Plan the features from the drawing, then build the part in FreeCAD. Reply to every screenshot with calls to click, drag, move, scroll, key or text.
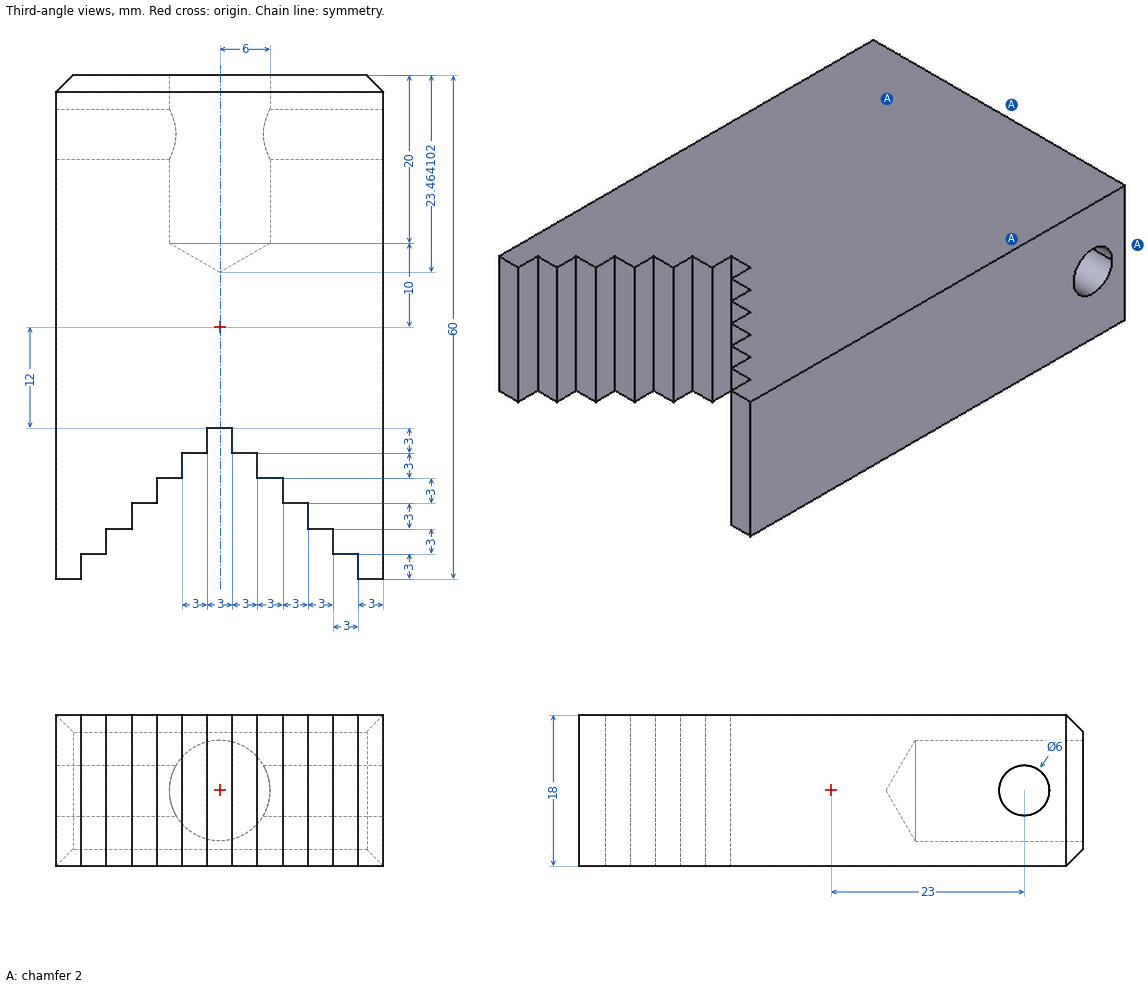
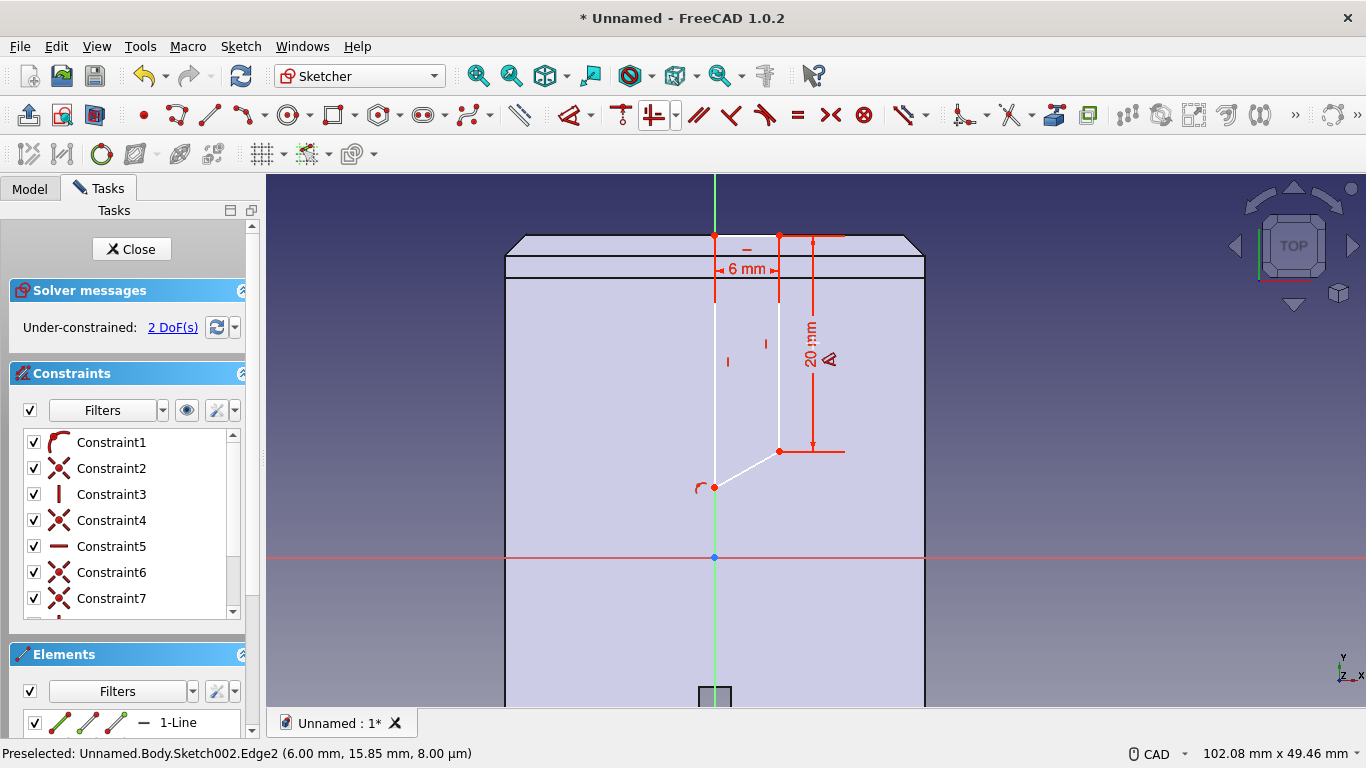
click(779, 452)
click(813, 505)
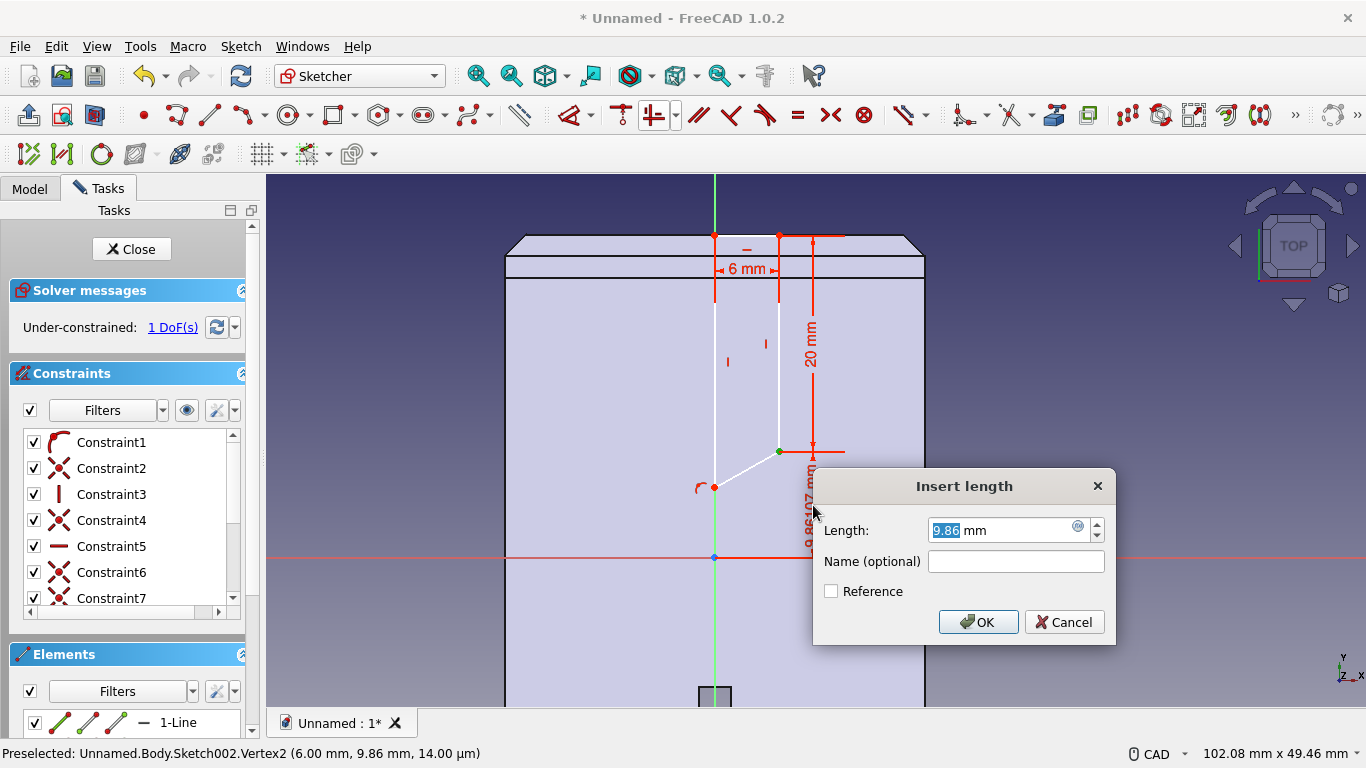
text(10)
key(Return)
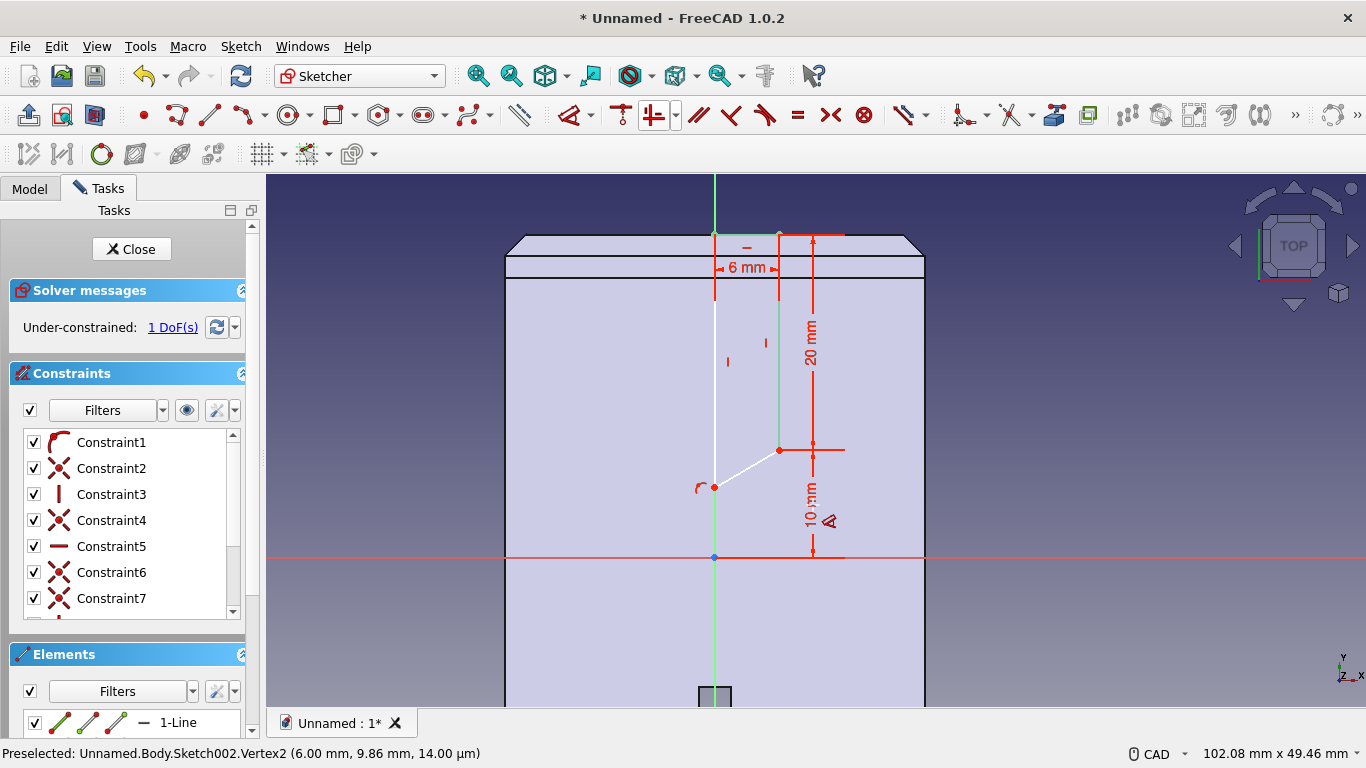
click(715, 311)
click(681, 361)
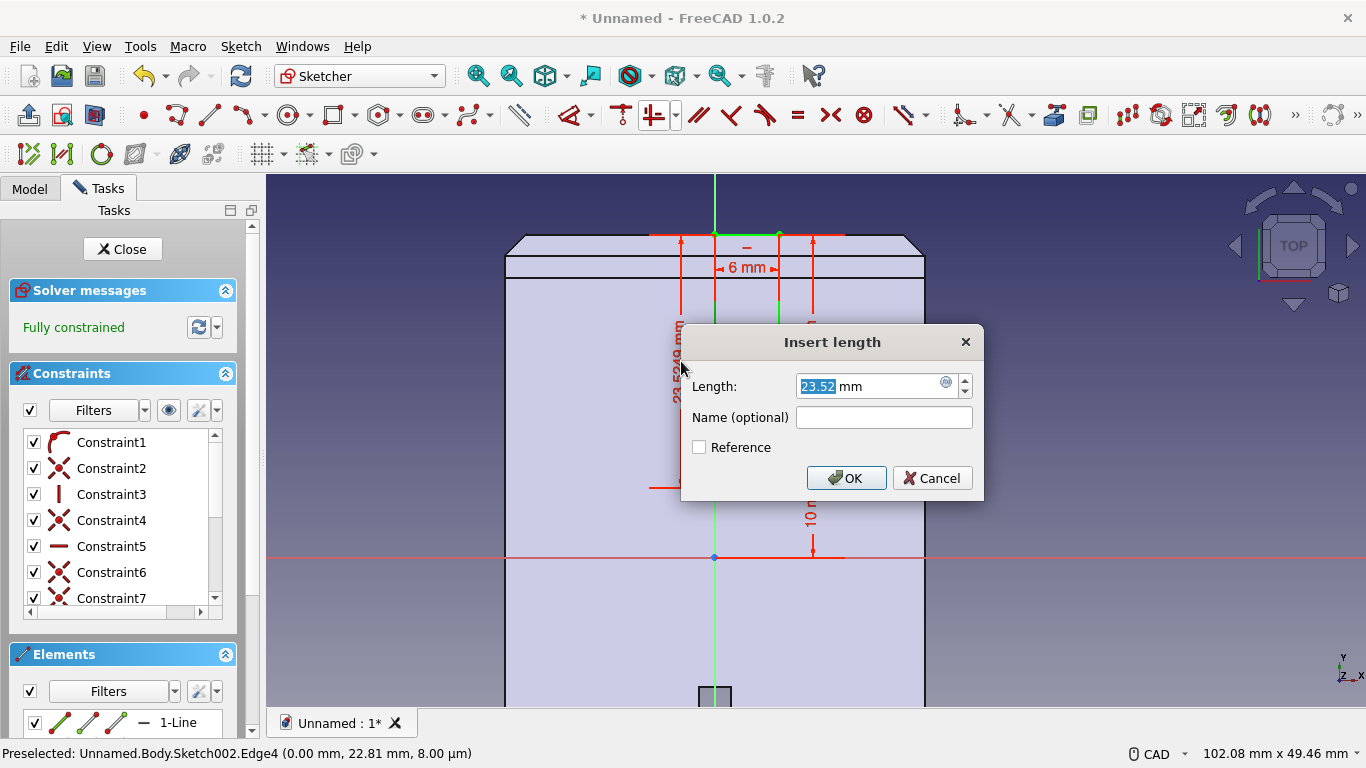
text(23.464102)
key(Return)
key(Escape)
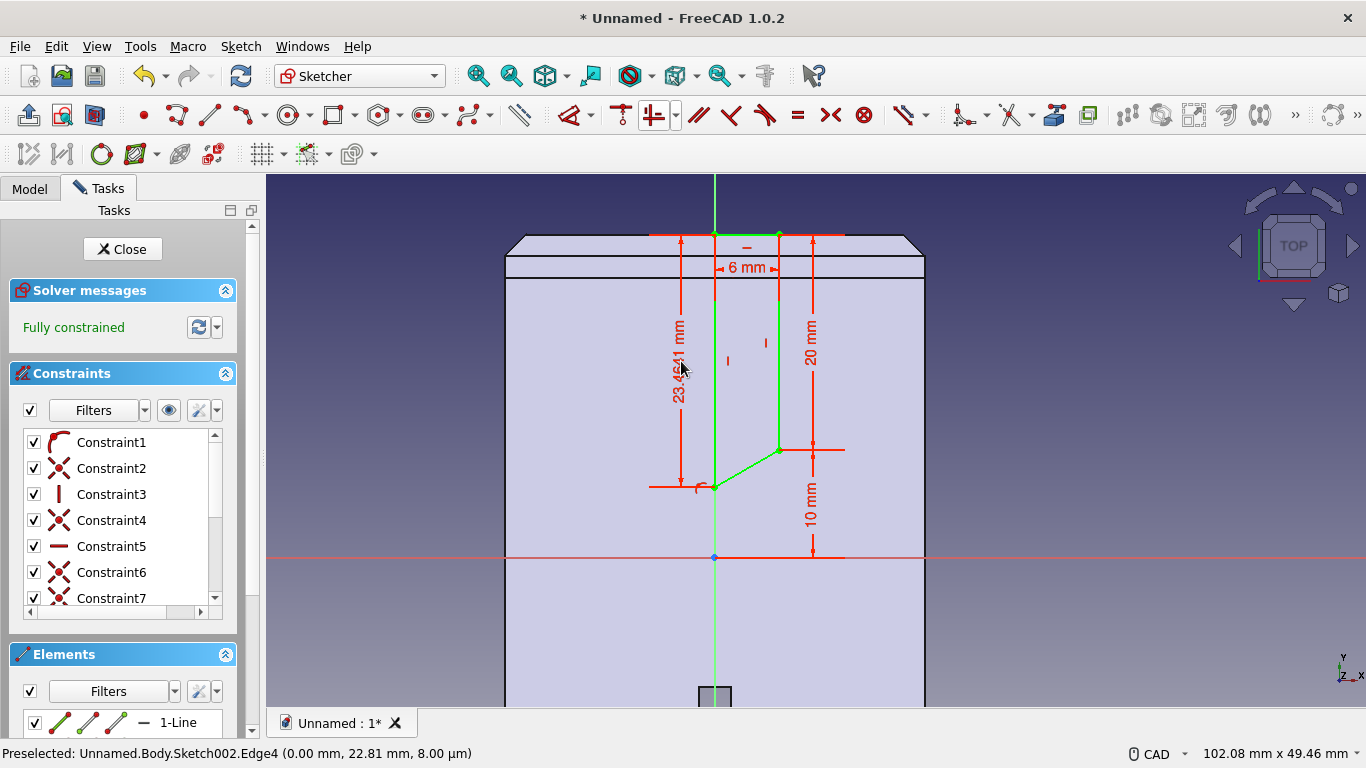
click(123, 249)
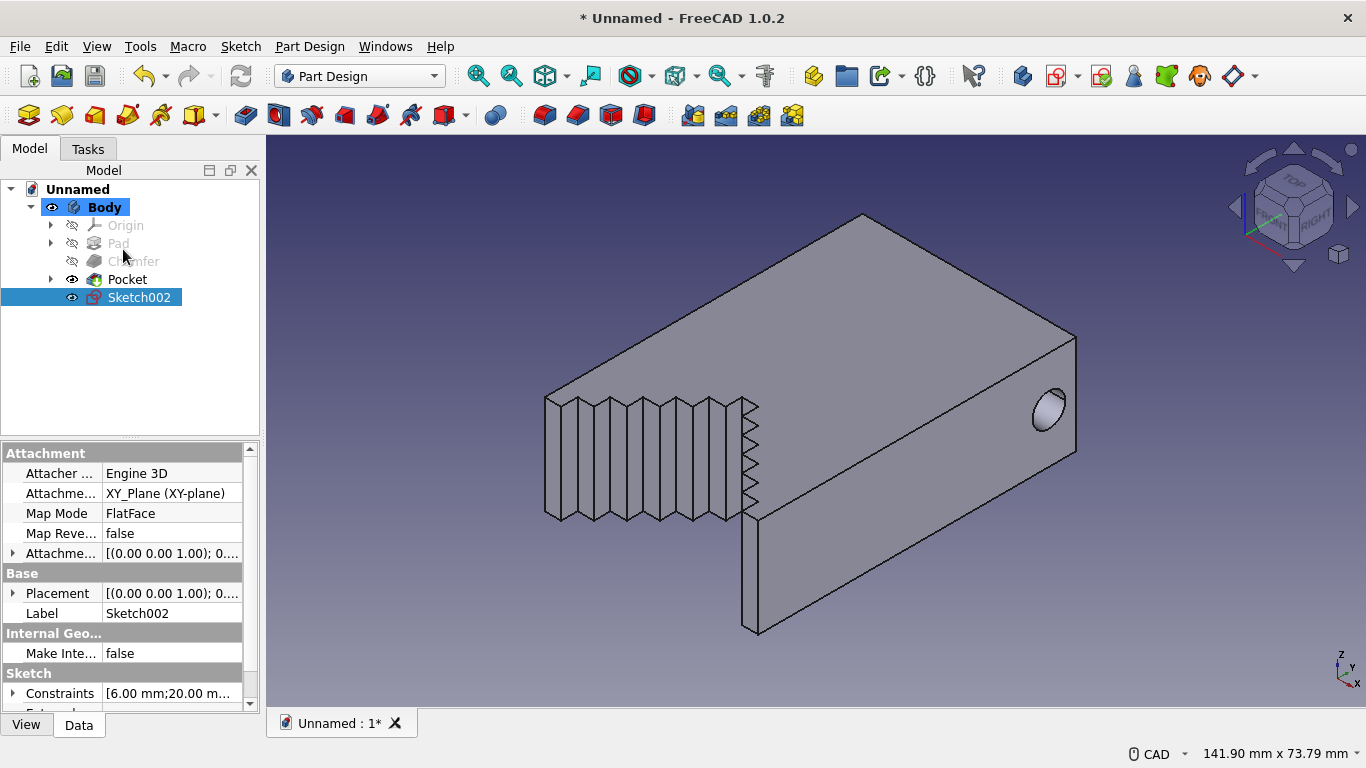
click(312, 116)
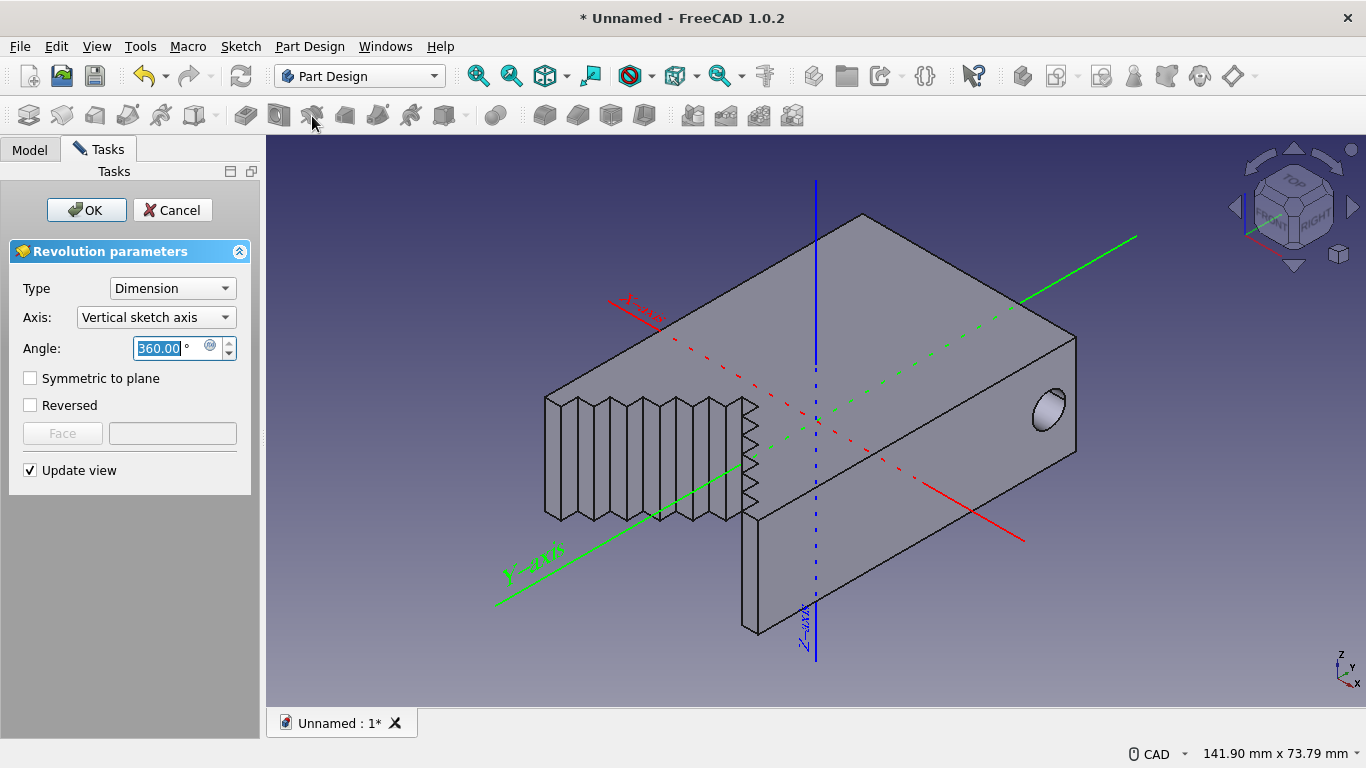
click(87, 210)